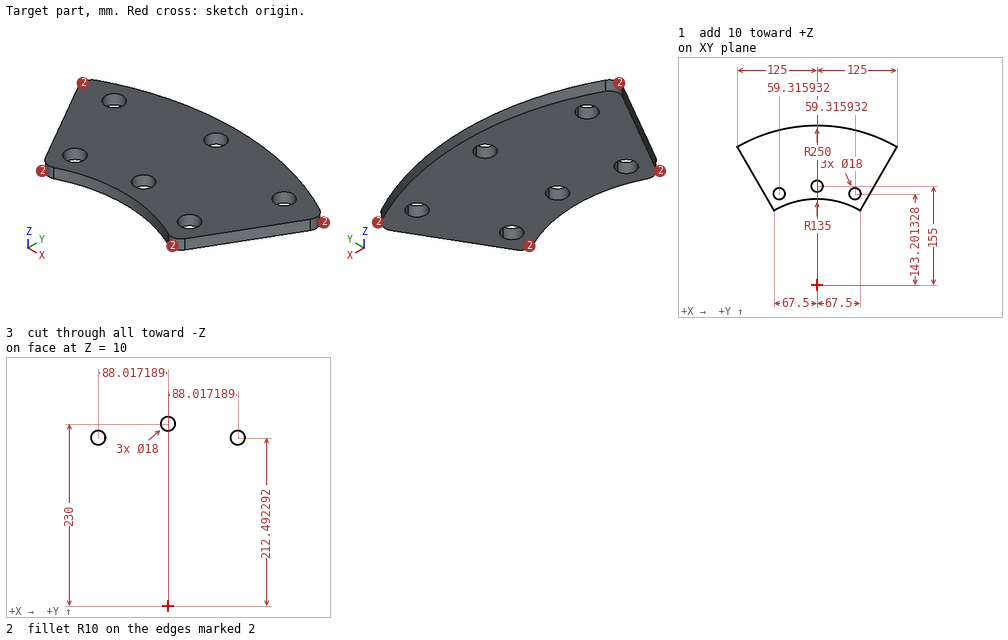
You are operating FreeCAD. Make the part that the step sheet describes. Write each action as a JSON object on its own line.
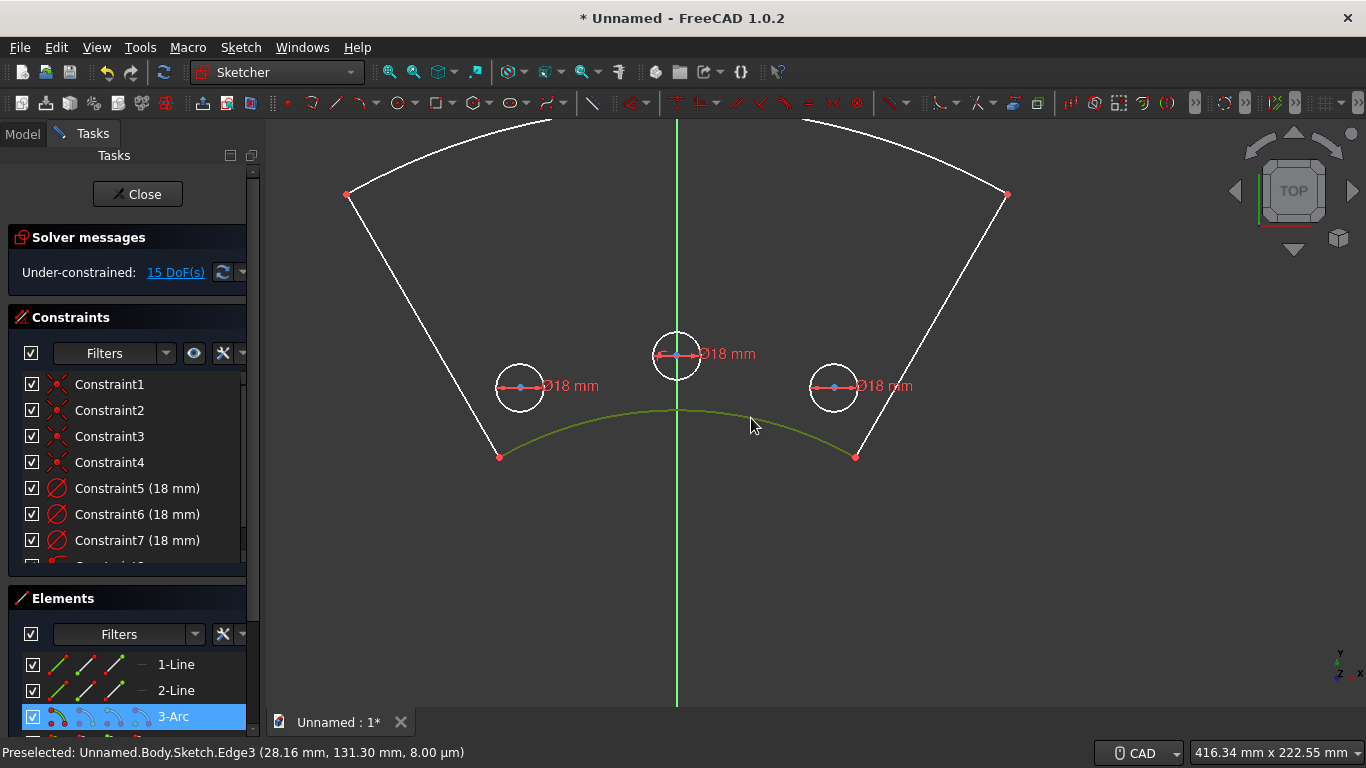
{"action": "scroll", "coordinate": [833, 387], "scroll_direction": "down", "scroll_amount": 3}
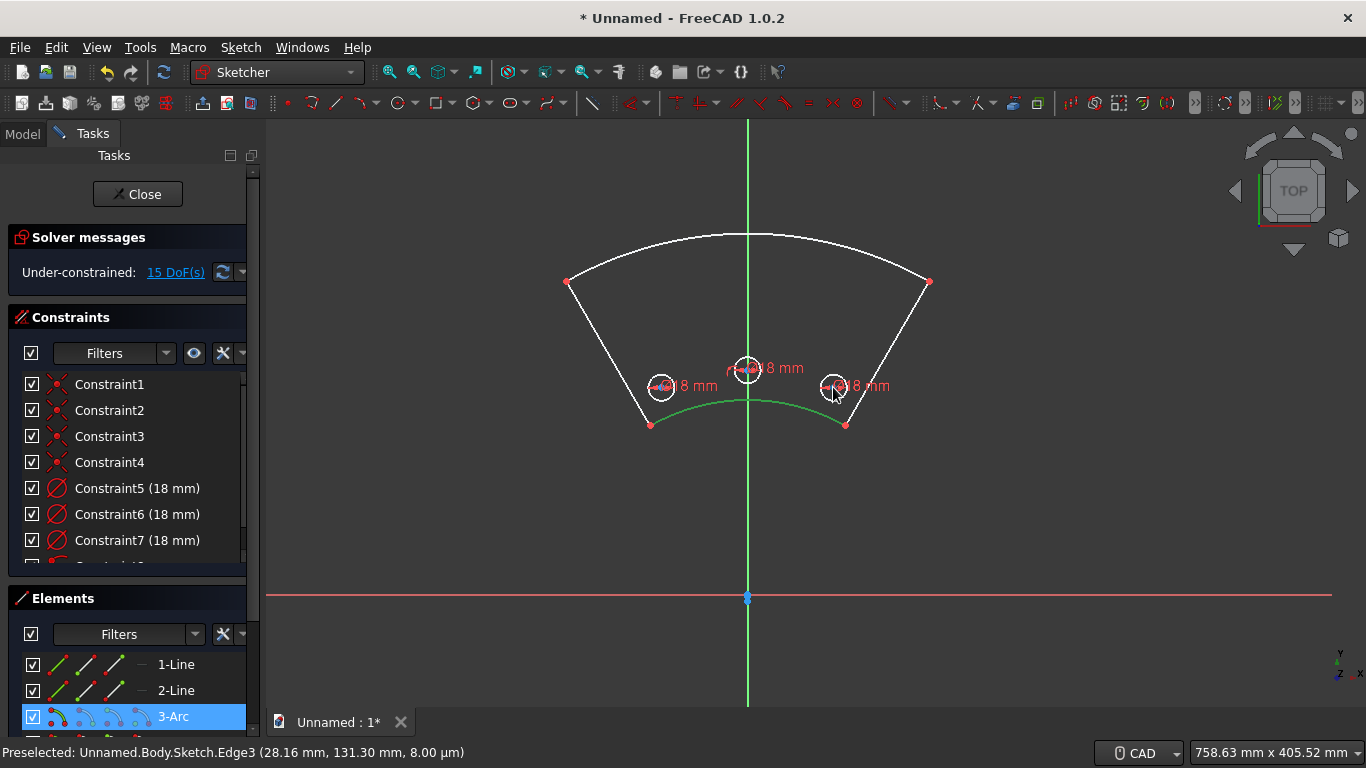
{"action": "left_click", "coordinate": [823, 241]}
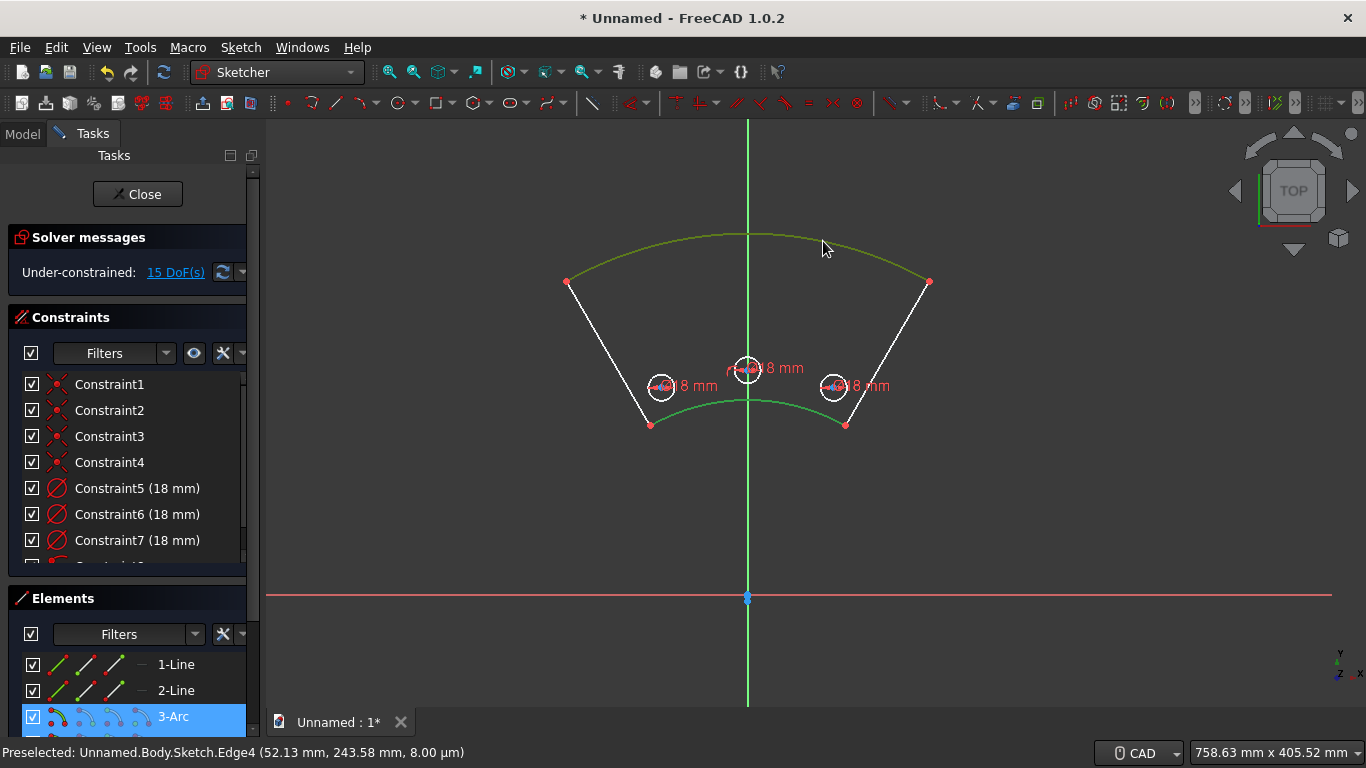
{"action": "left_click", "coordinate": [676, 104]}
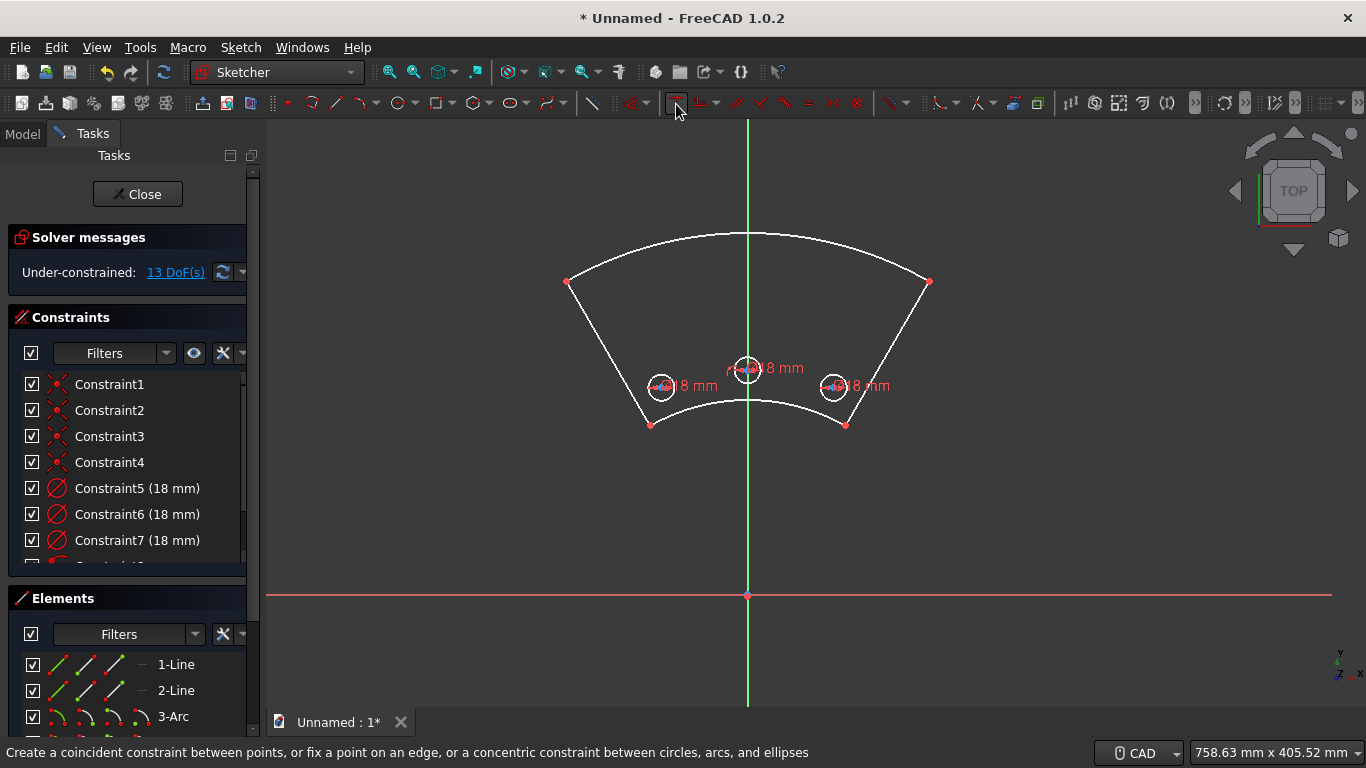
{"action": "scroll", "coordinate": [748, 596], "scroll_direction": "up", "scroll_amount": 6}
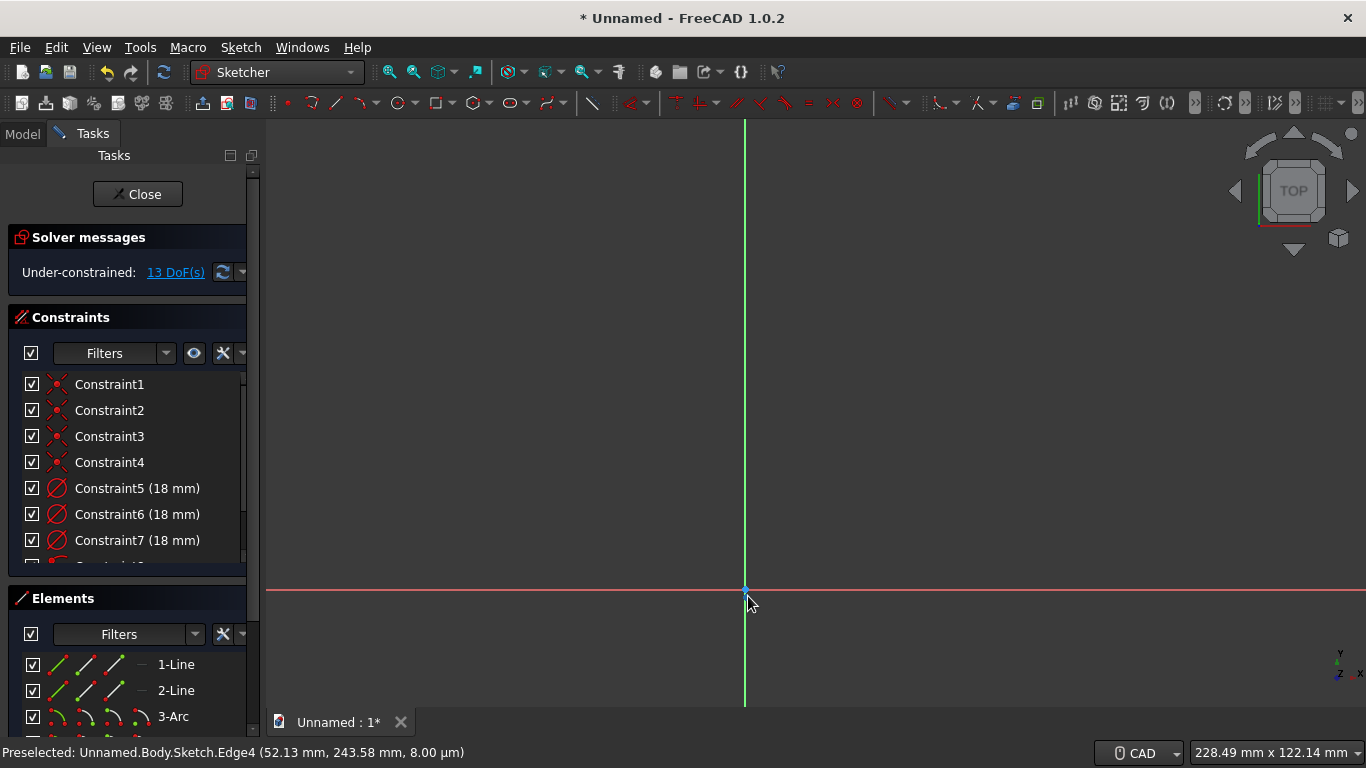
{"action": "left_click_drag", "start_coordinate": [735, 580], "coordinate": [756, 607]}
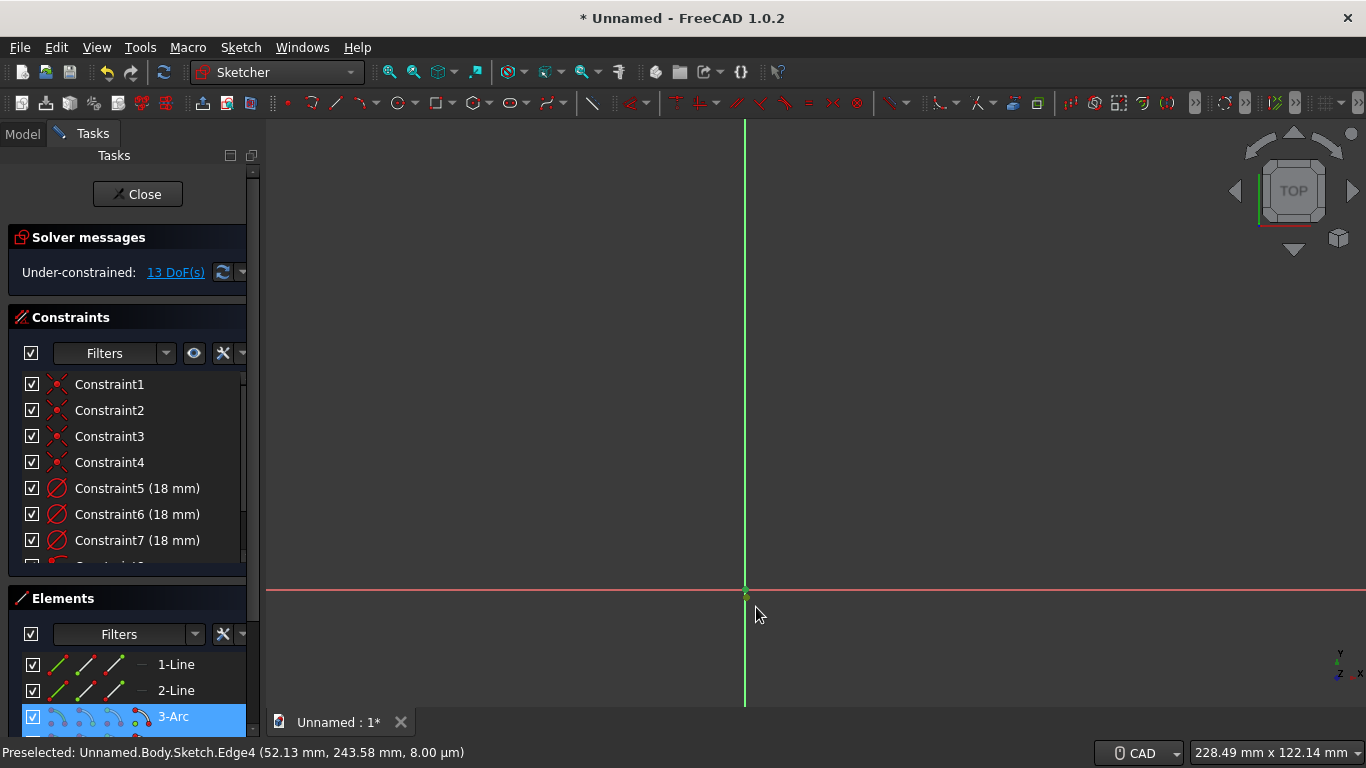
{"action": "left_click", "coordinate": [676, 104]}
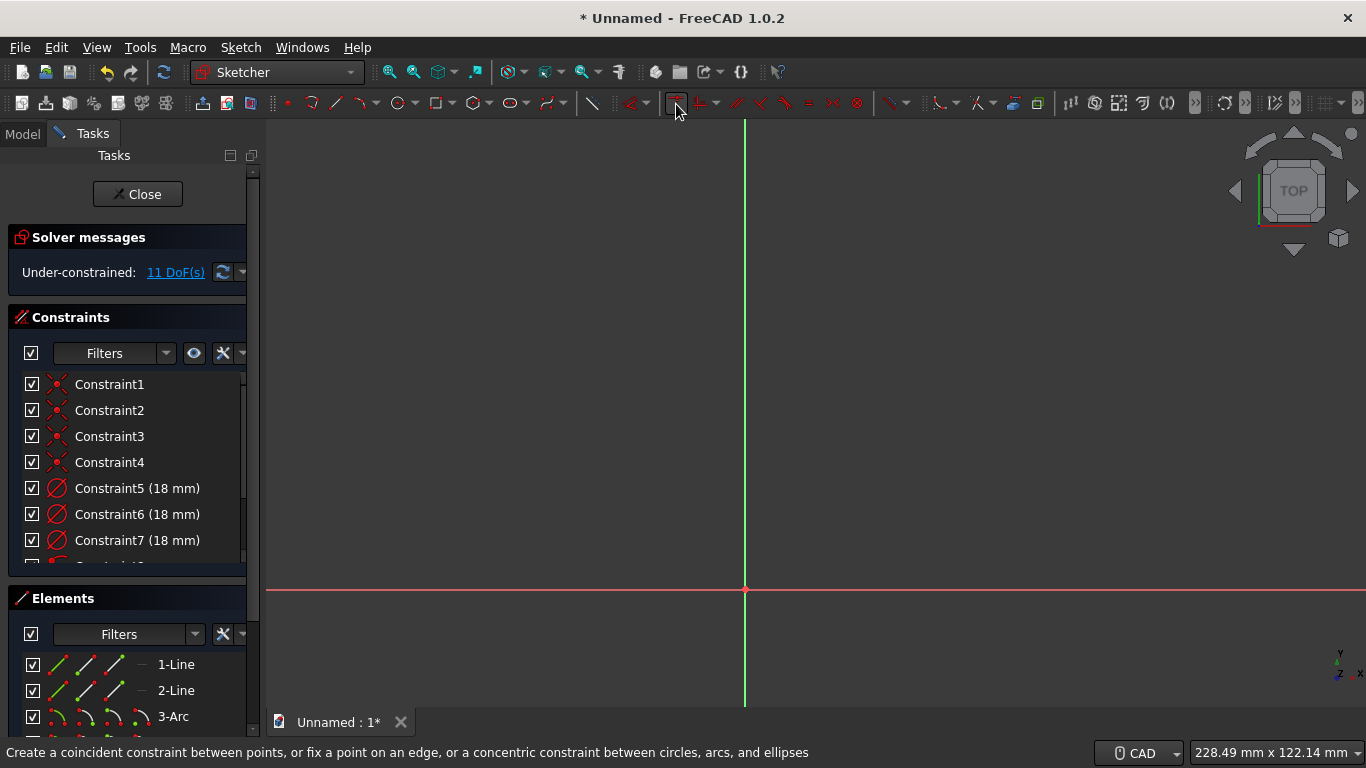
{"action": "scroll", "coordinate": [748, 596], "scroll_direction": "down", "scroll_amount": 6}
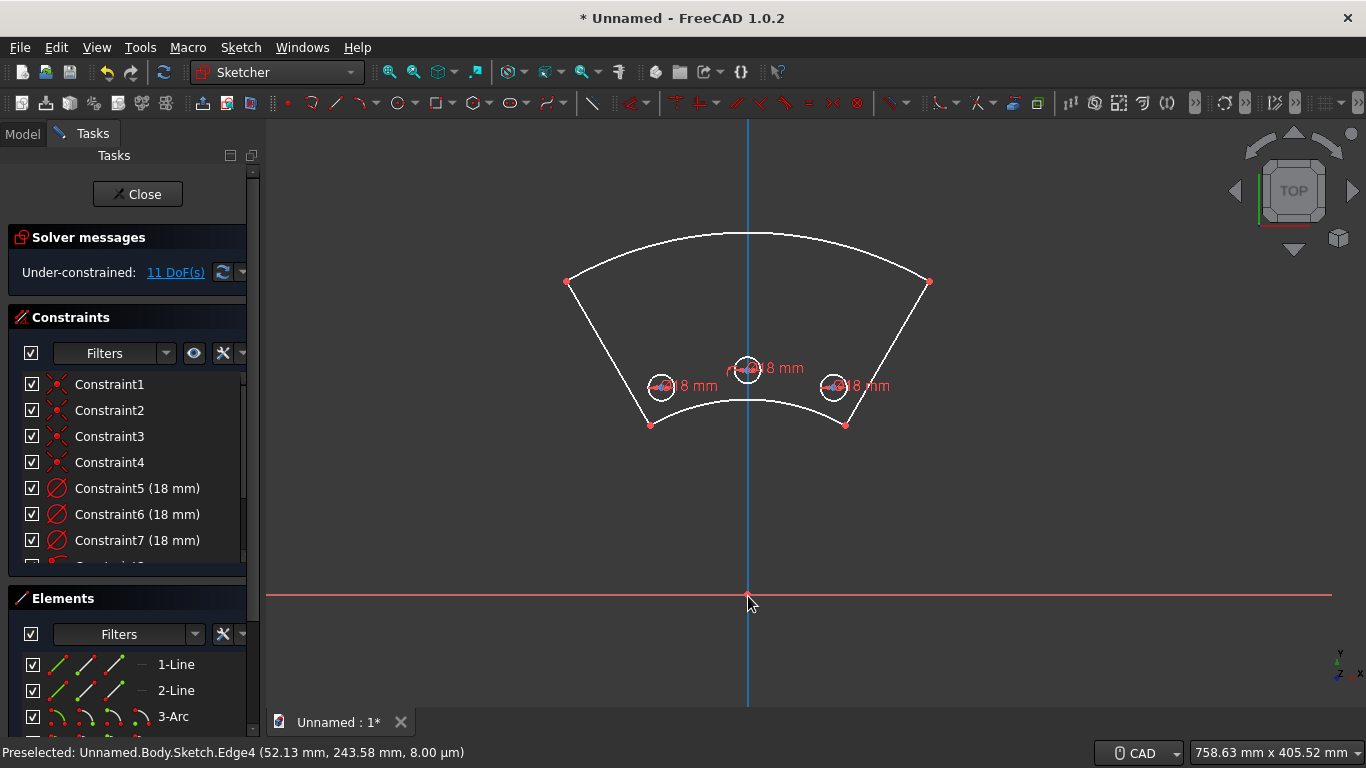
{"action": "left_click", "coordinate": [834, 388]}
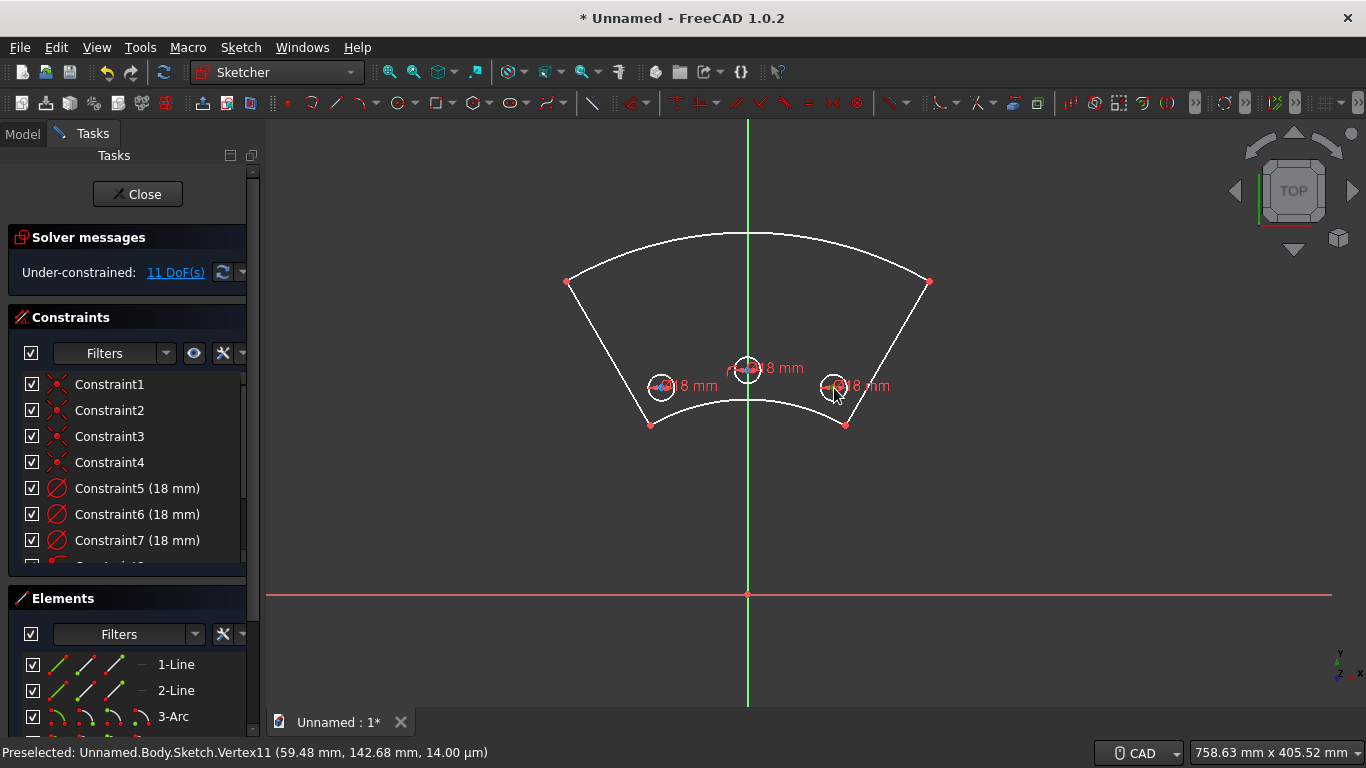
{"action": "left_click", "coordinate": [661, 388]}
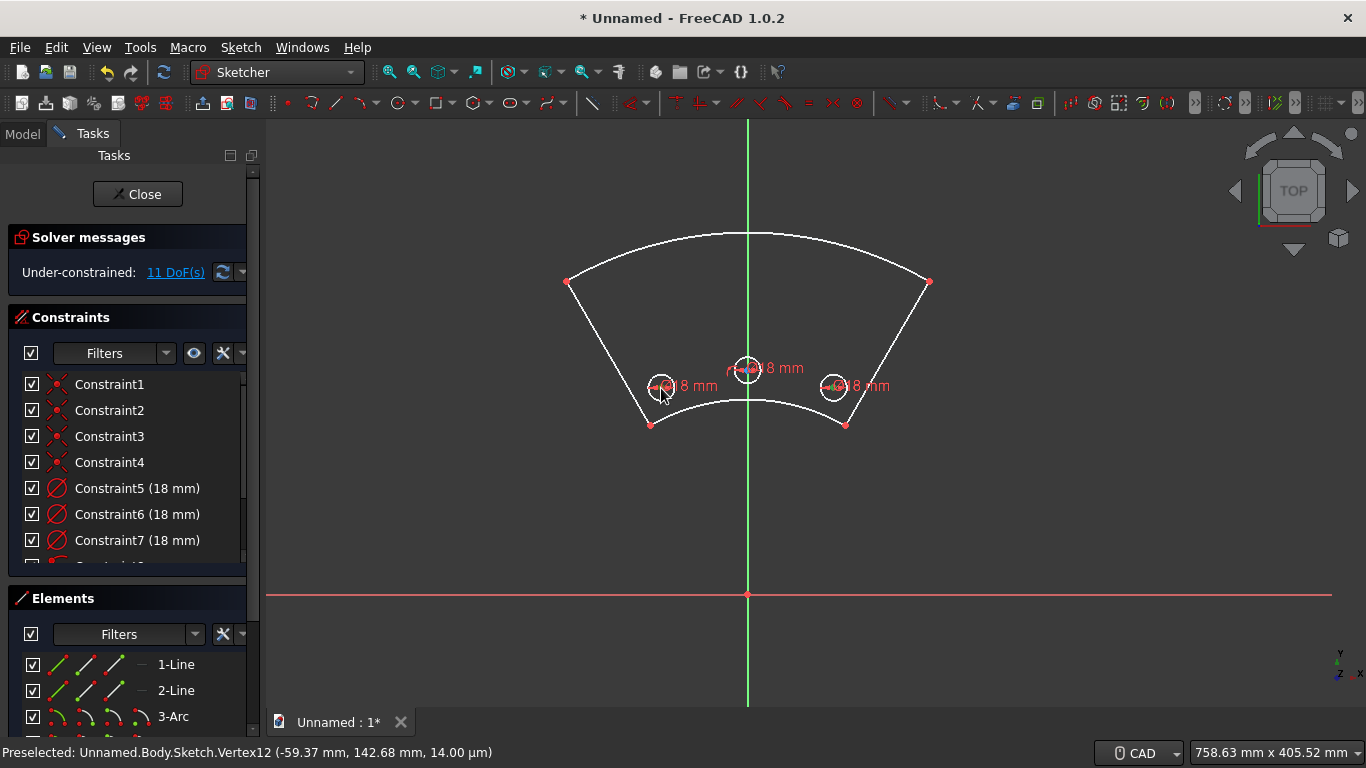
{"action": "key", "text": "h"}